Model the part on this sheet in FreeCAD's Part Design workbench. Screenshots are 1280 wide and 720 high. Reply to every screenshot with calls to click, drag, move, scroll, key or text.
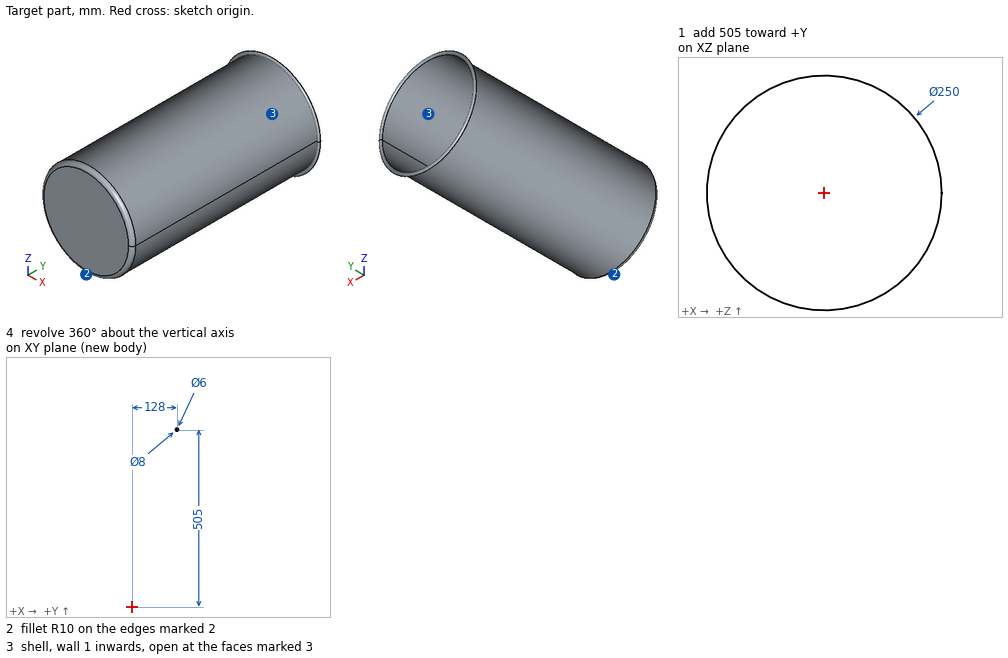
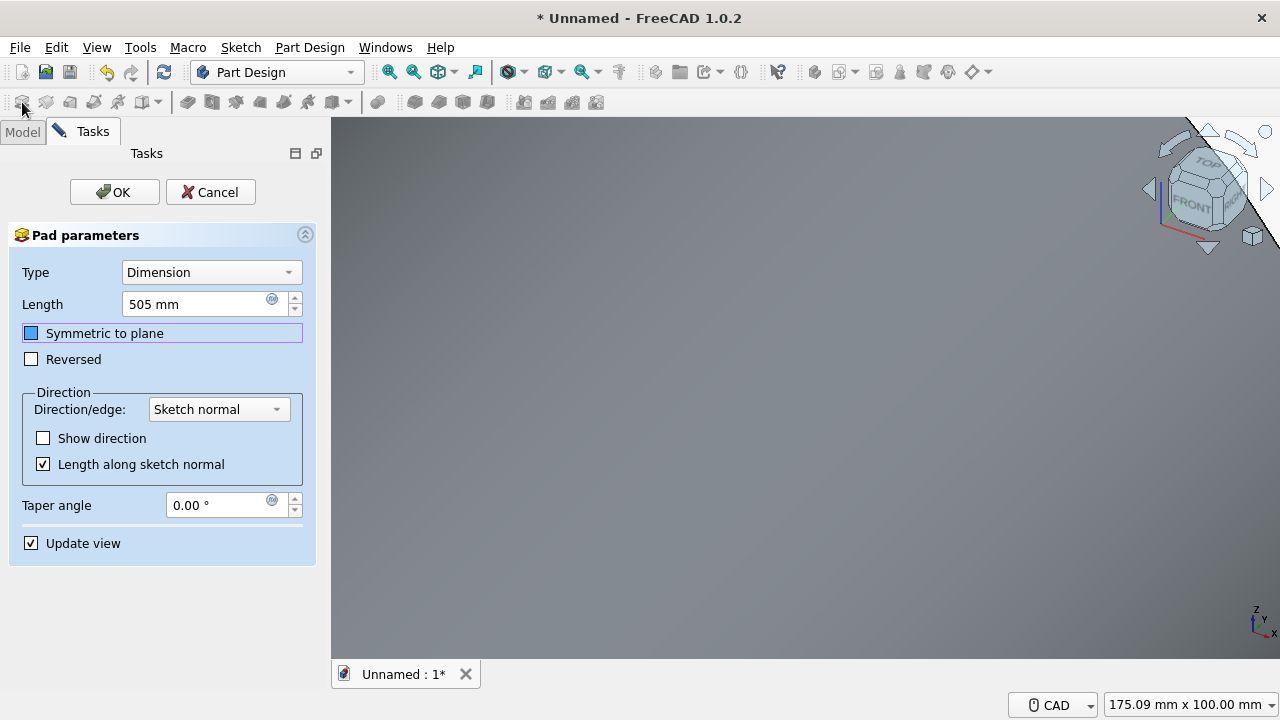
click(30, 359)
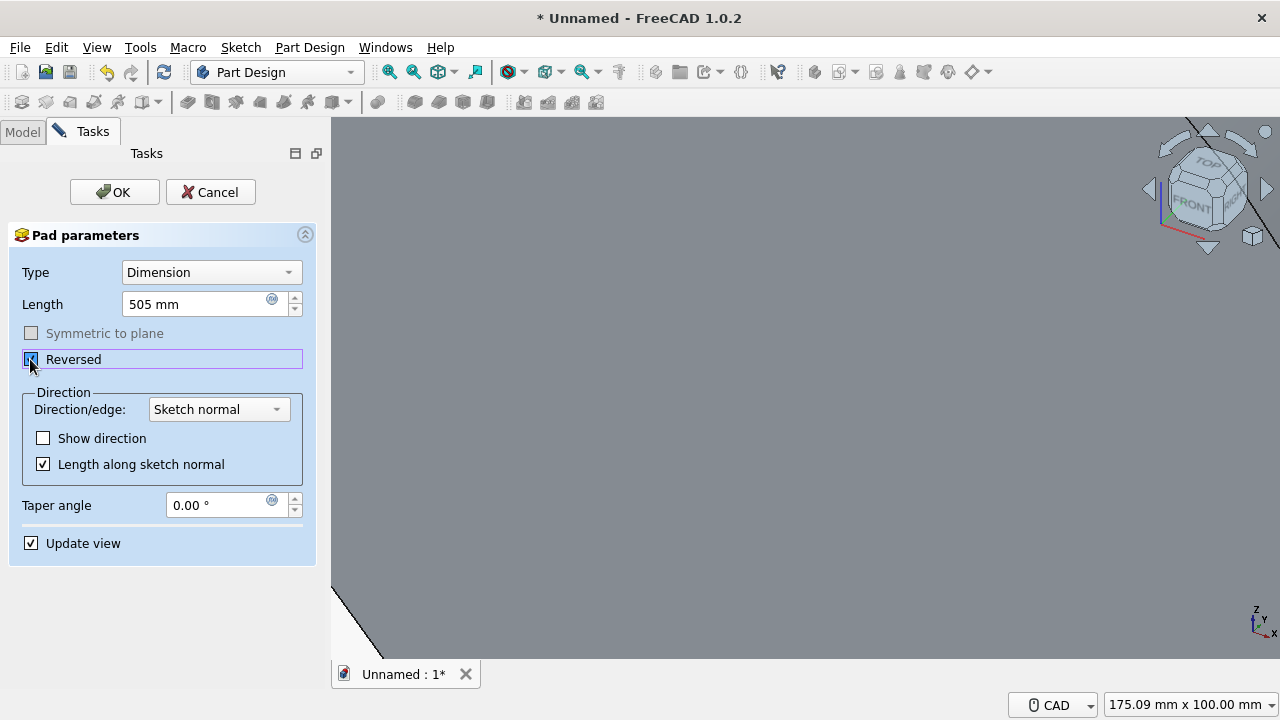
click(115, 192)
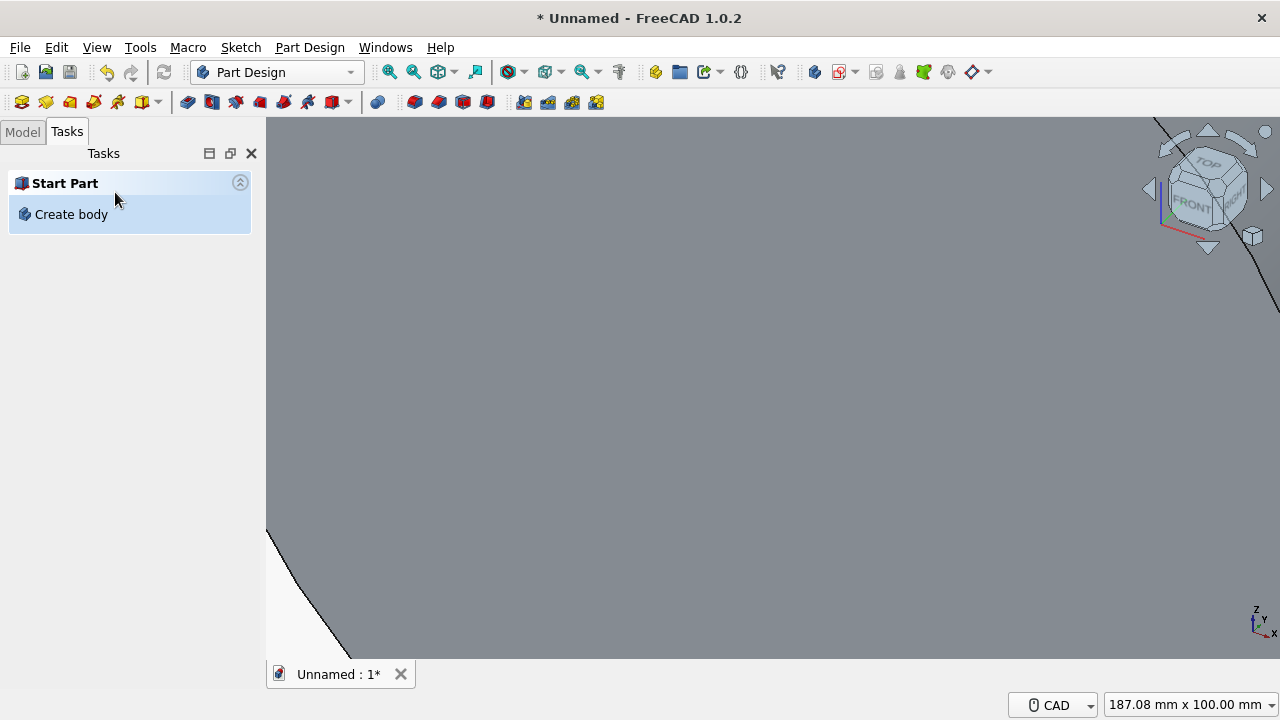
click(390, 72)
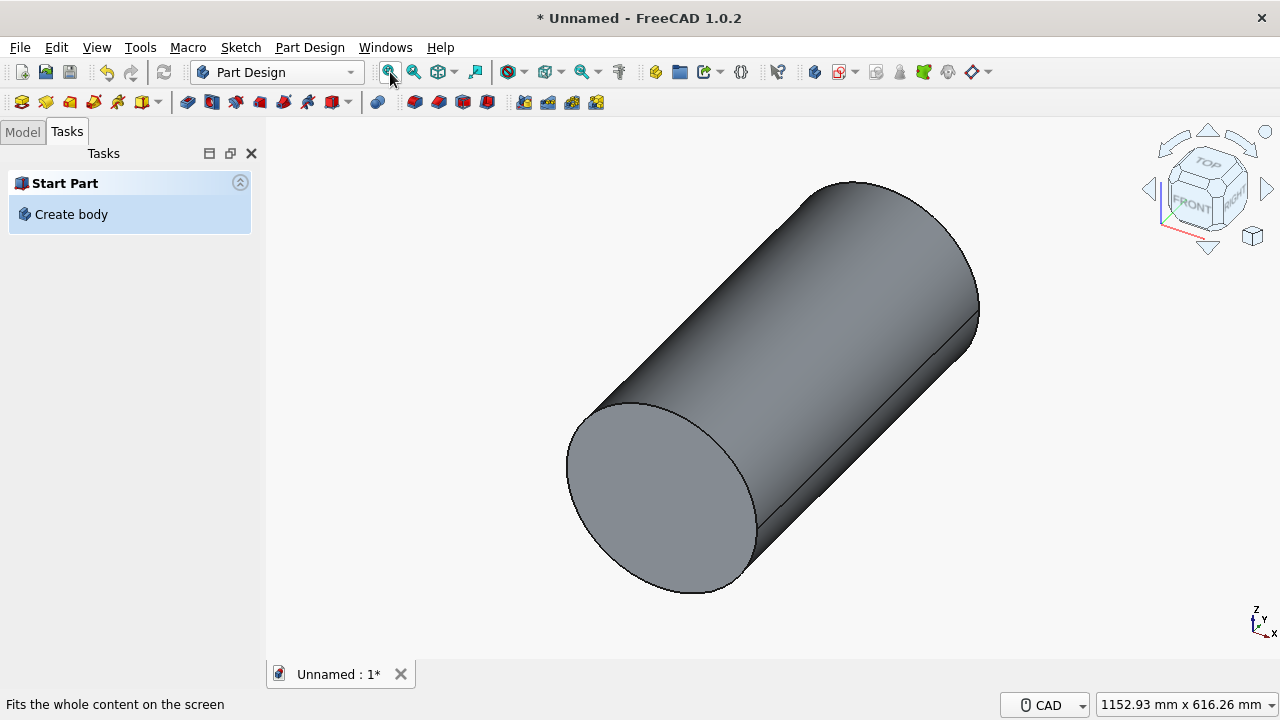
click(632, 402)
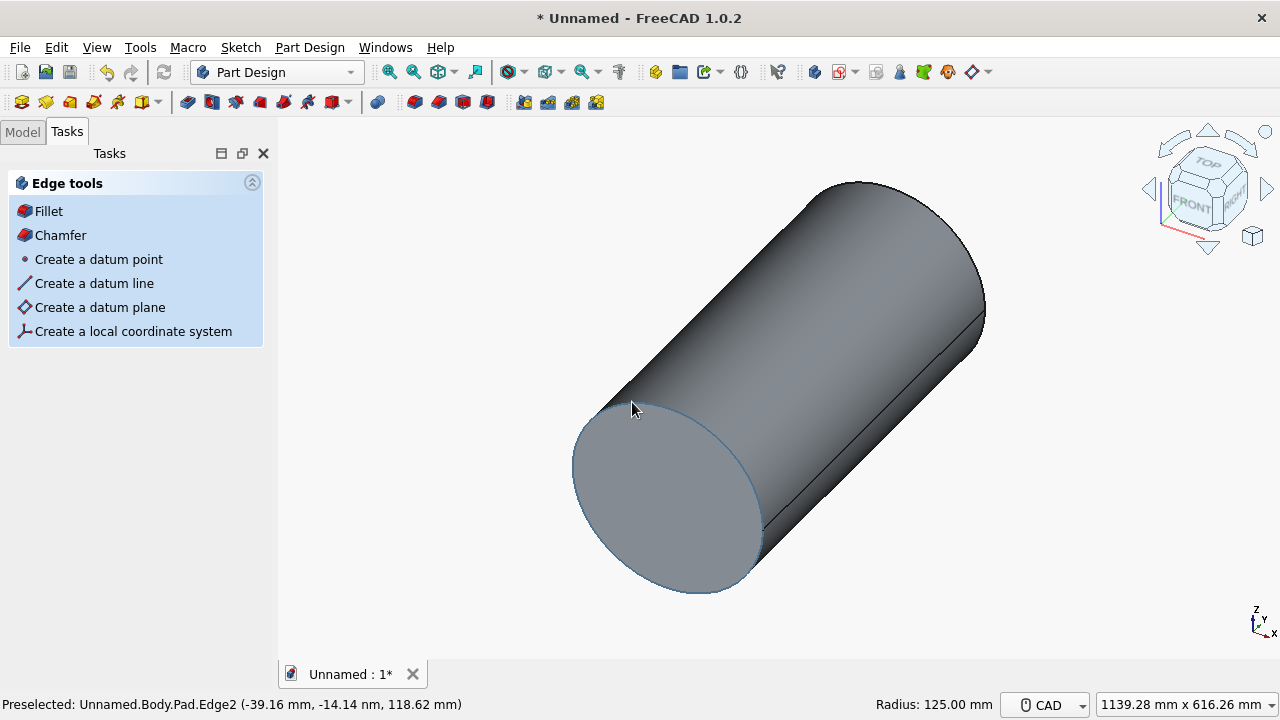
click(416, 102)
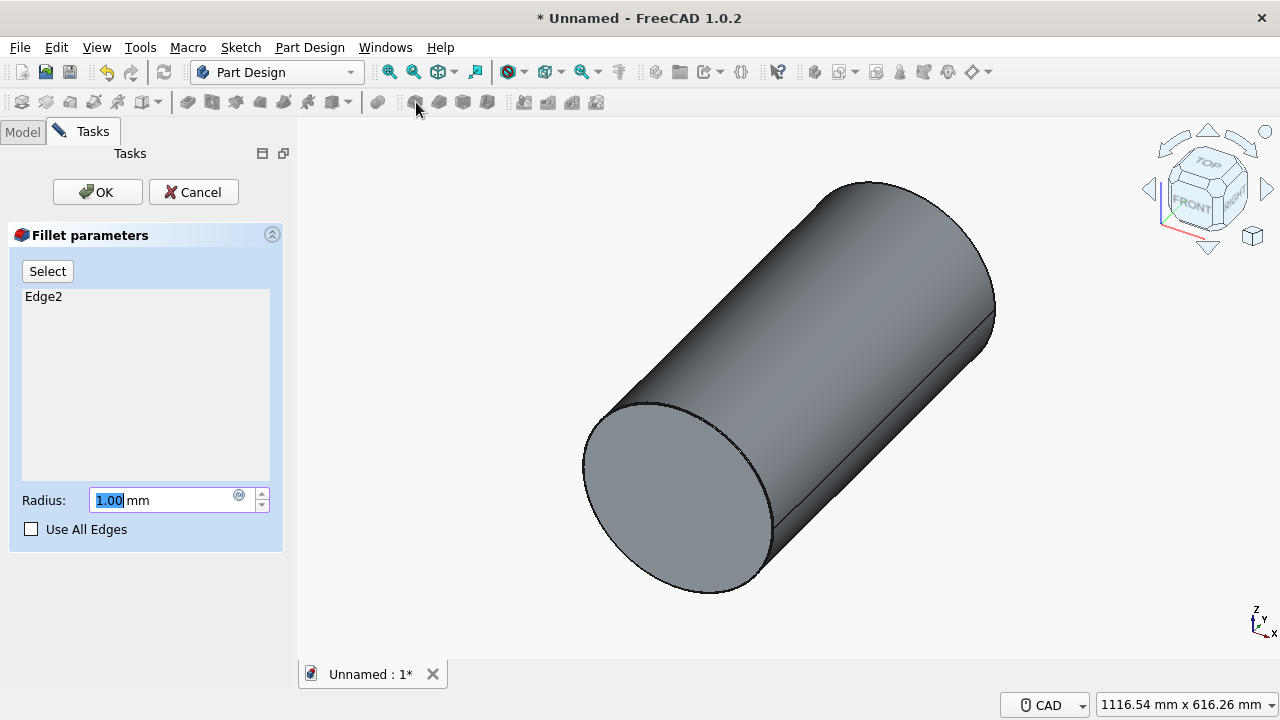
text(10)
key(Tab)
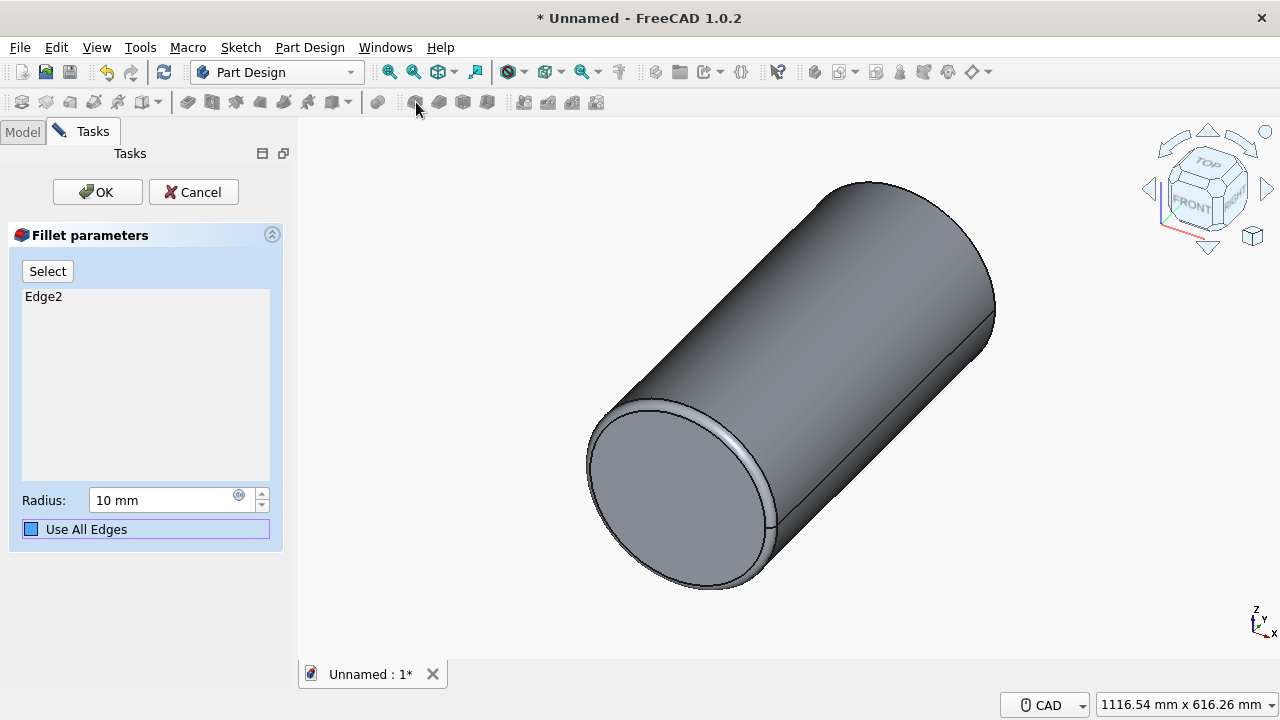
click(98, 192)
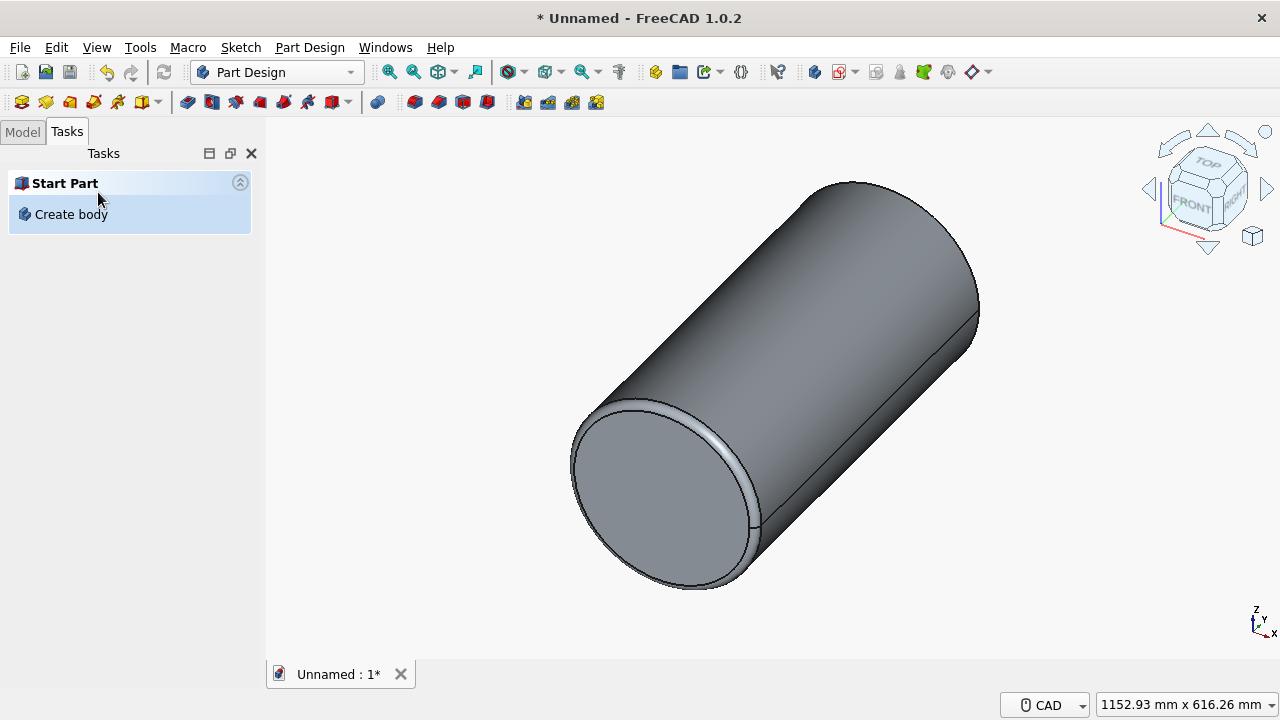
key(0)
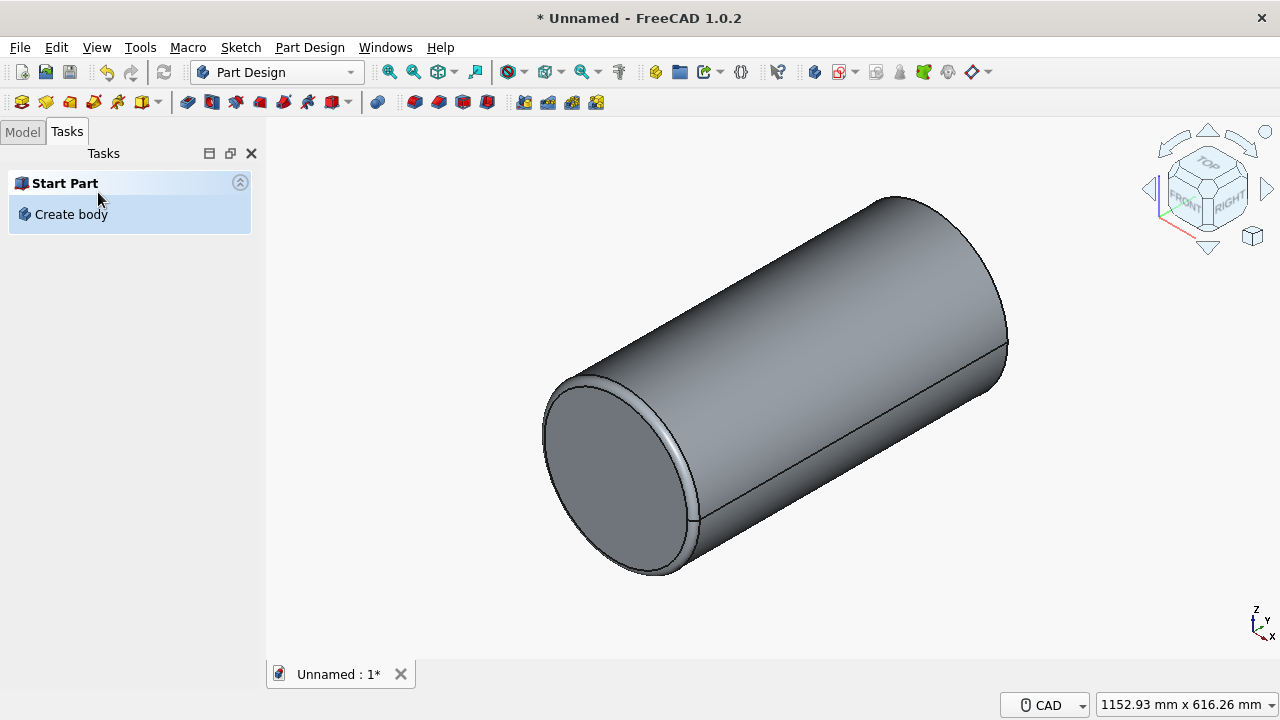
key(2)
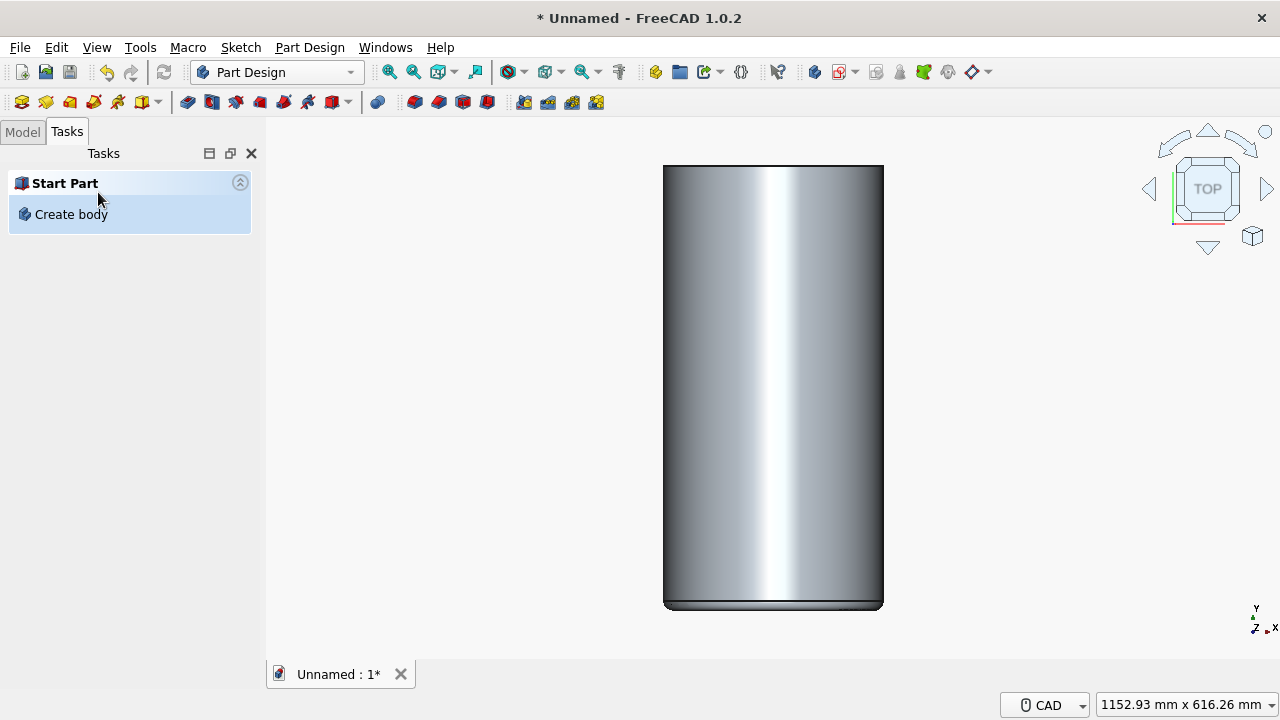
key(1)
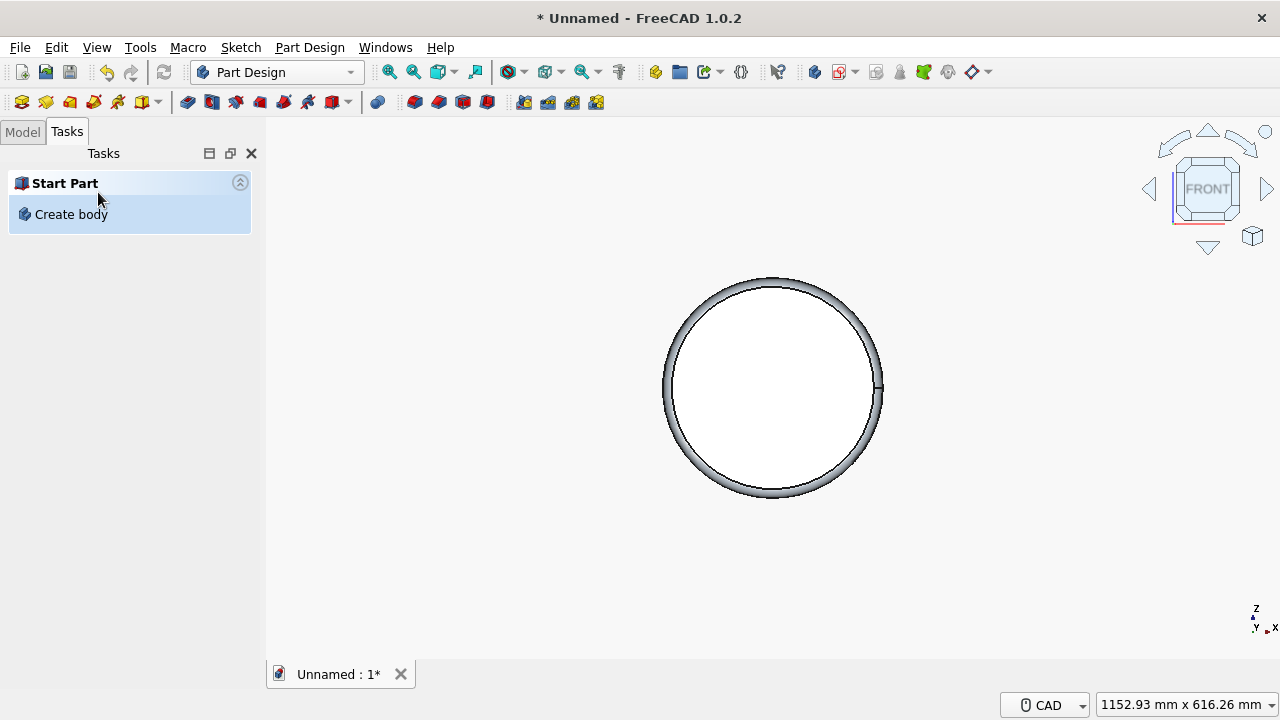
click(390, 72)